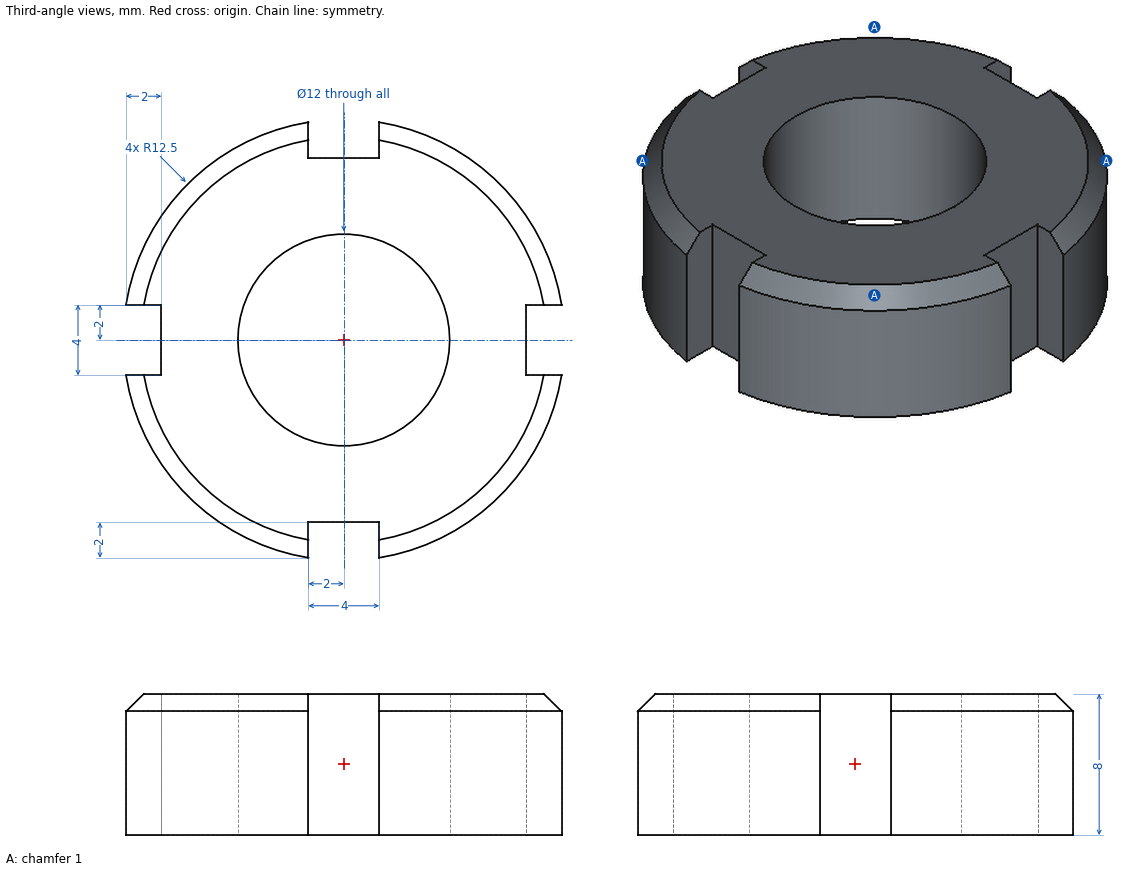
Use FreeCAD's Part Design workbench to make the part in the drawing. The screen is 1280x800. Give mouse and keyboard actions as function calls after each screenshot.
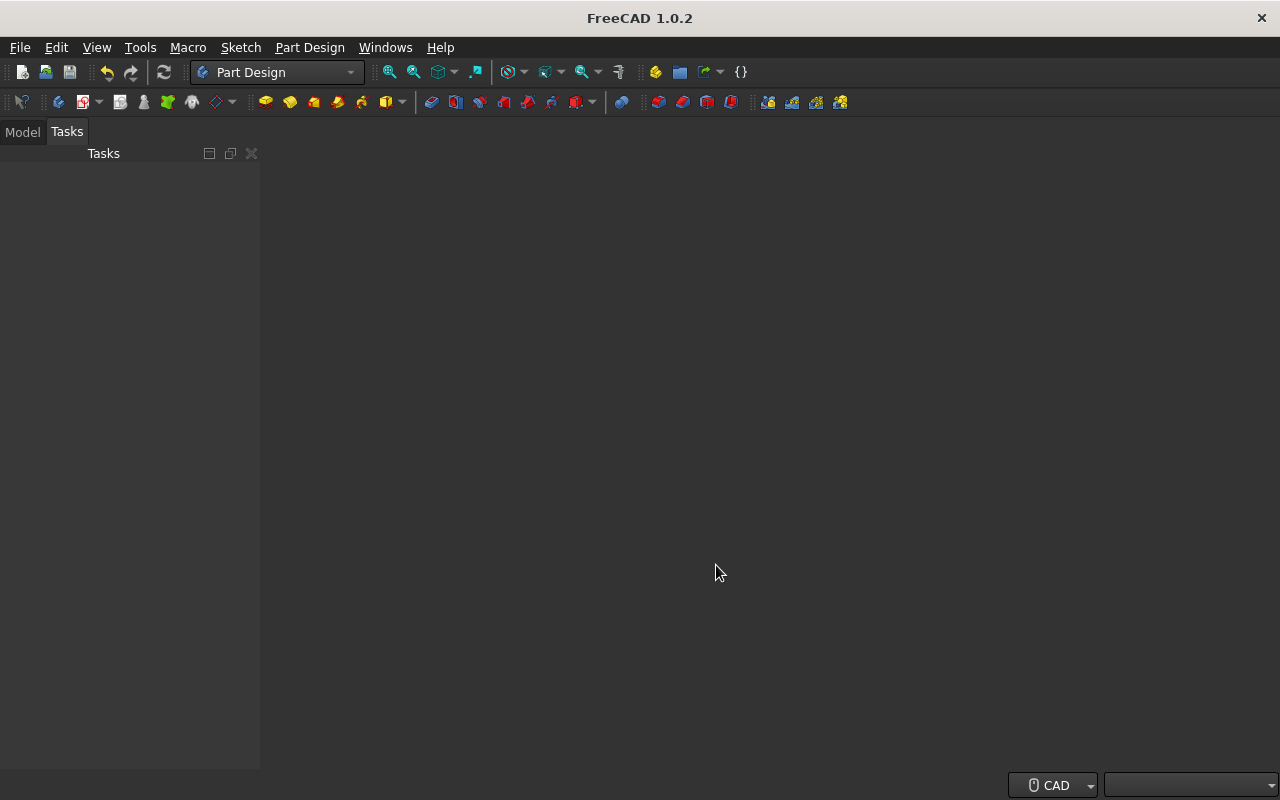
click(22, 72)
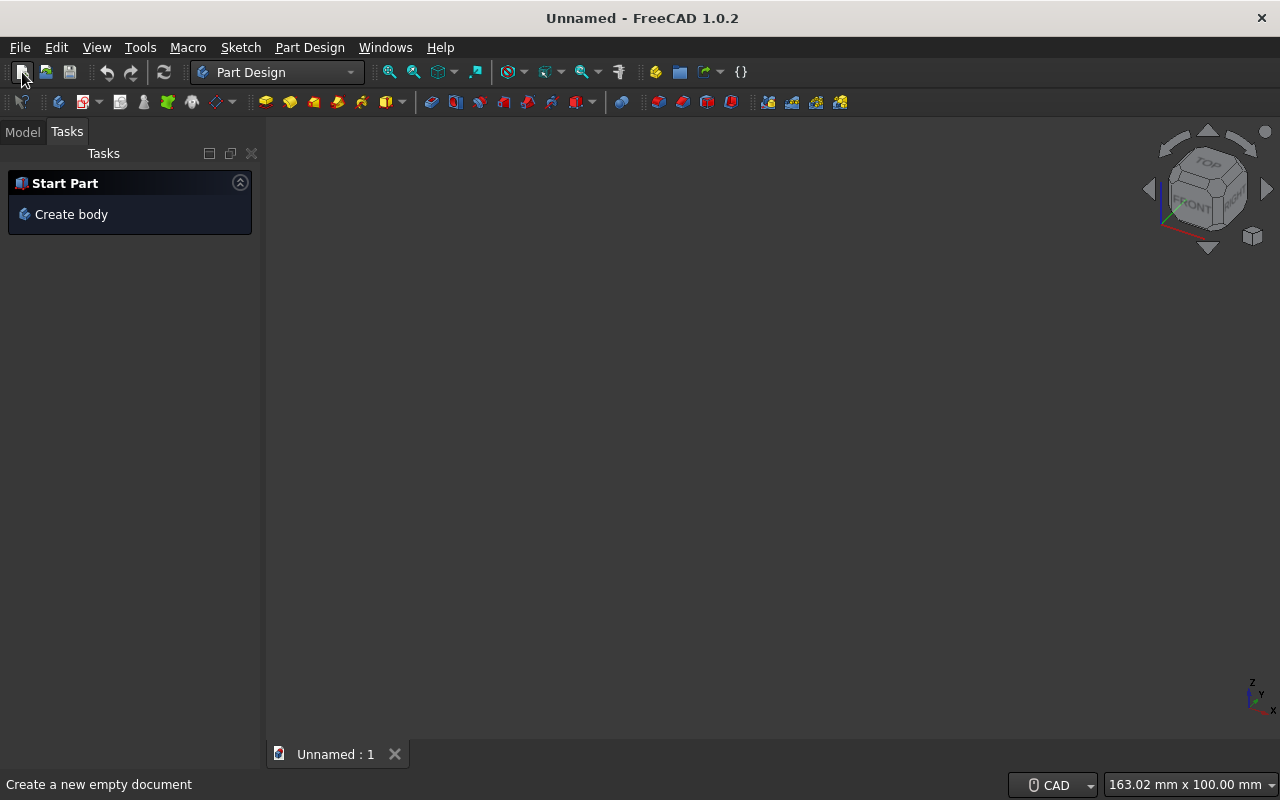
click(84, 102)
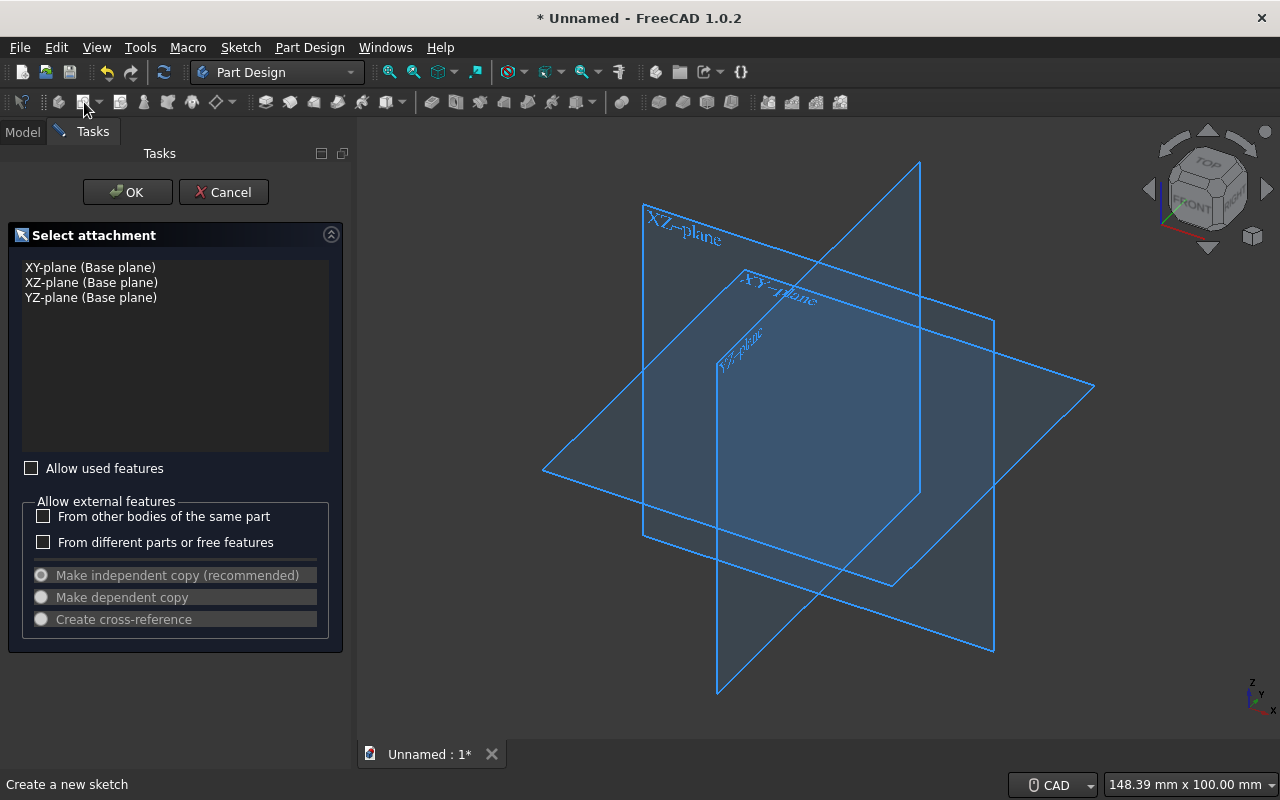
click(82, 268)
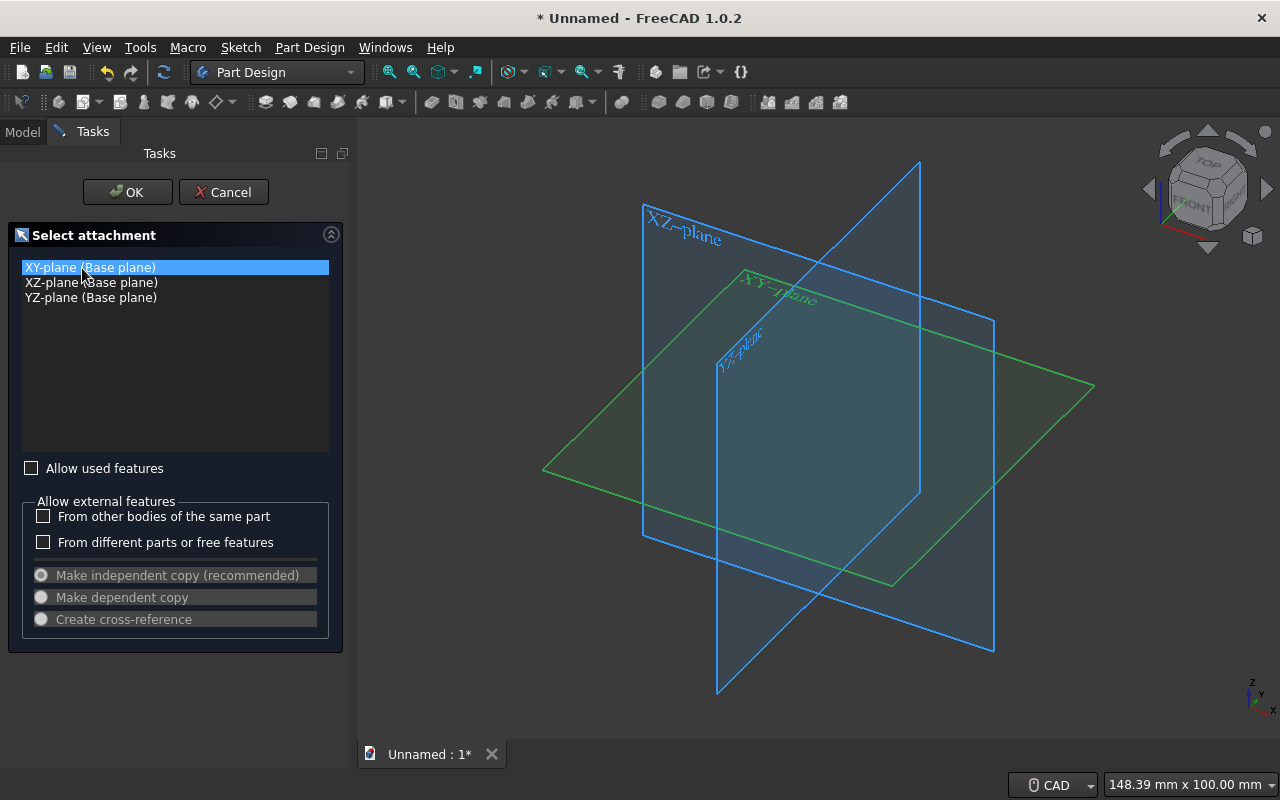
click(128, 192)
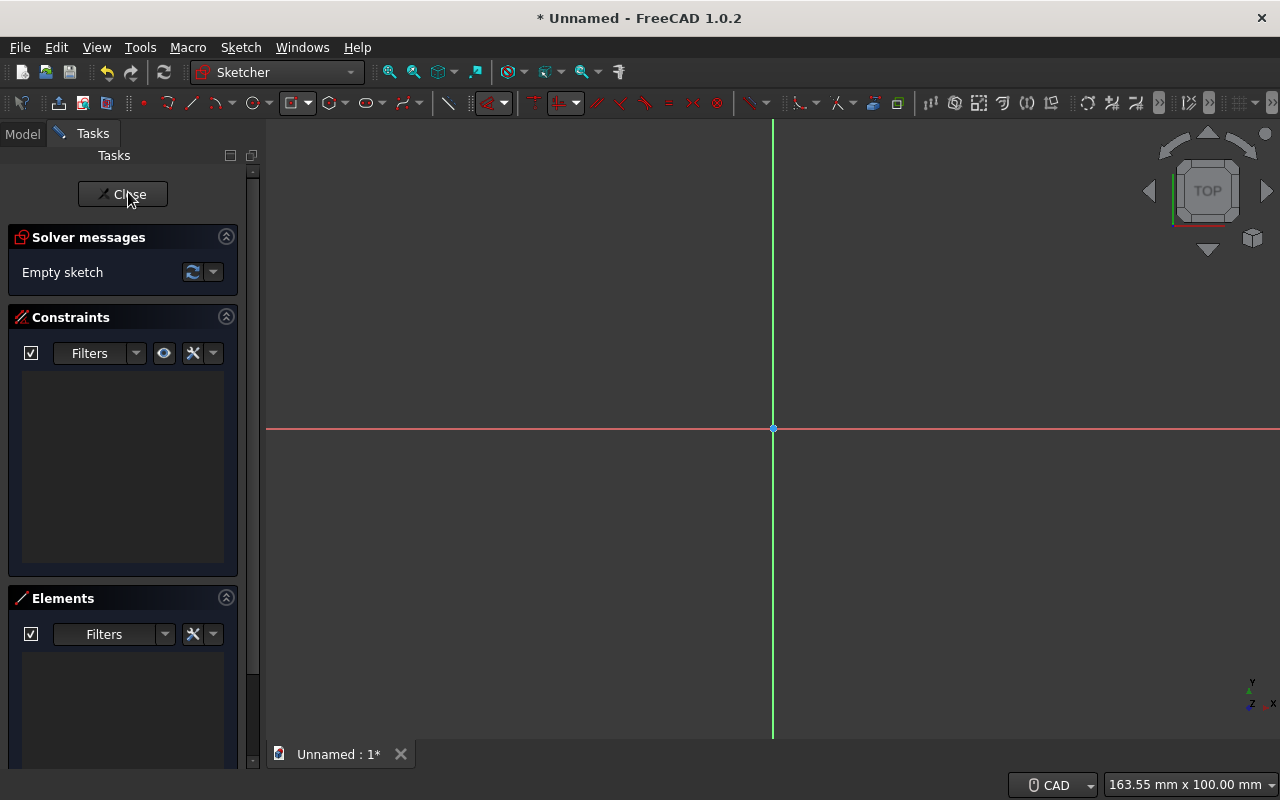
scroll(813, 429, up, 5)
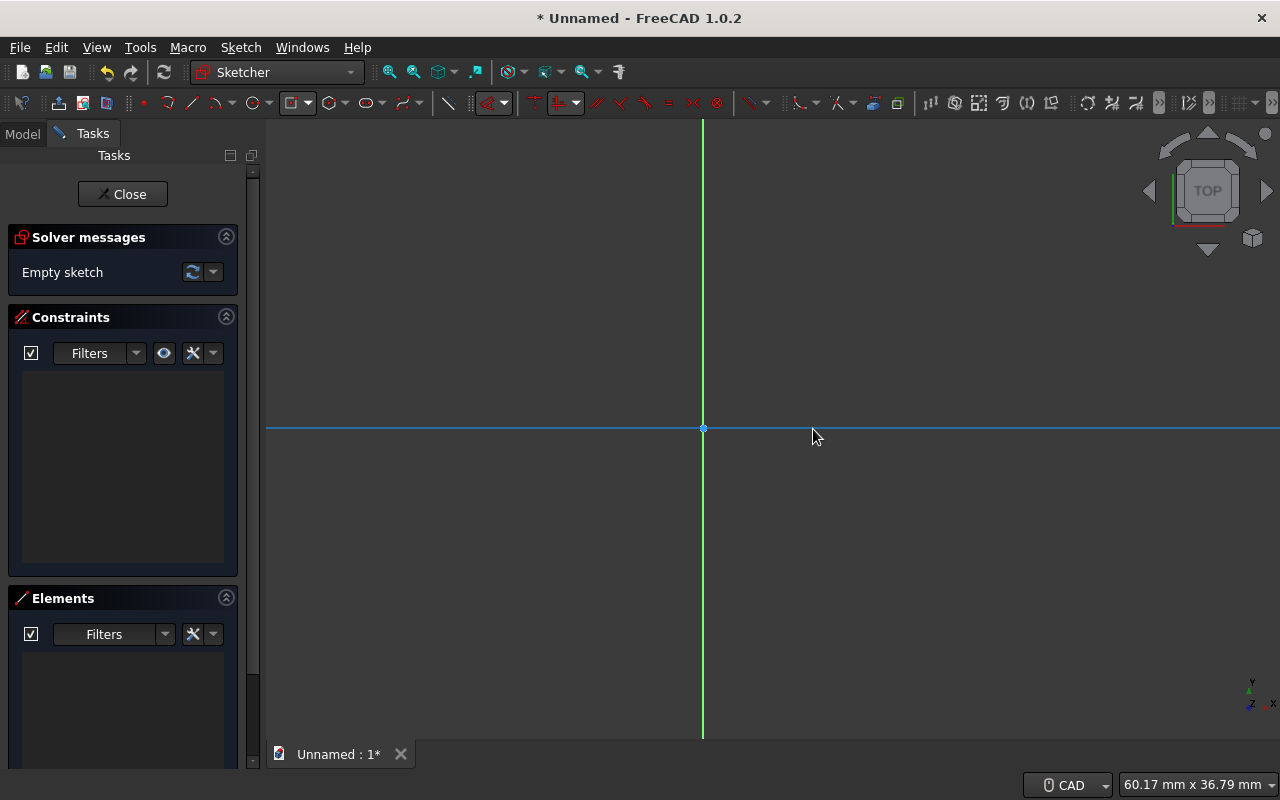
key(g)
key(m)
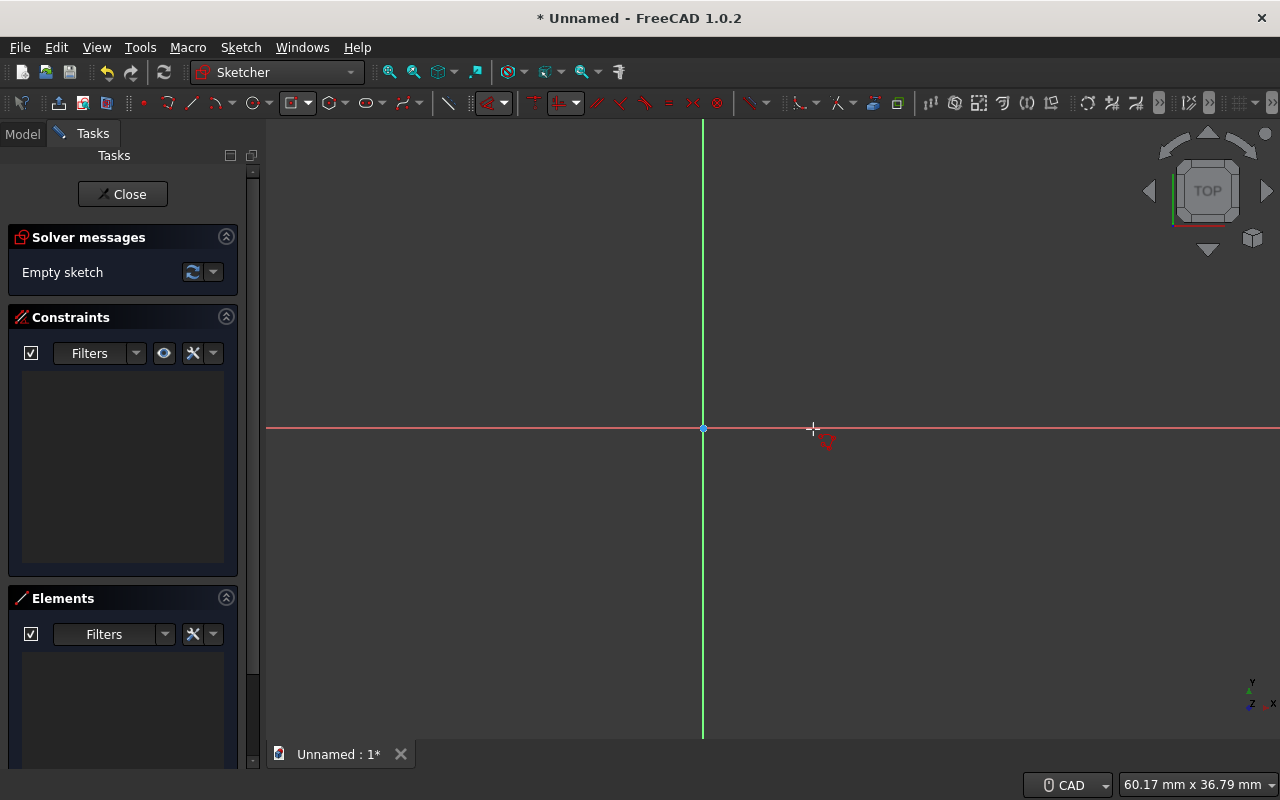
click(495, 394)
click(529, 394)
click(529, 462)
click(495, 462)
right_click(495, 462)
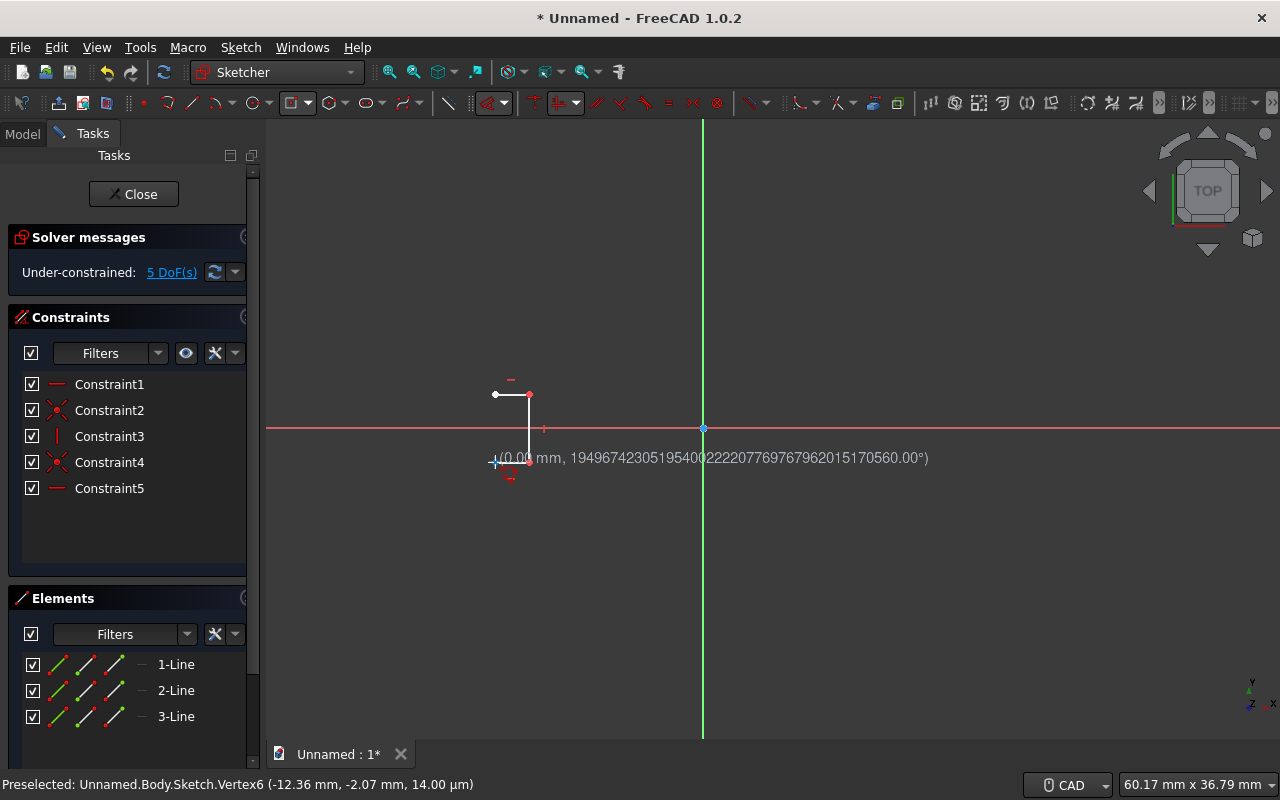
click(670, 636)
click(670, 602)
click(737, 602)
click(737, 636)
right_click(737, 636)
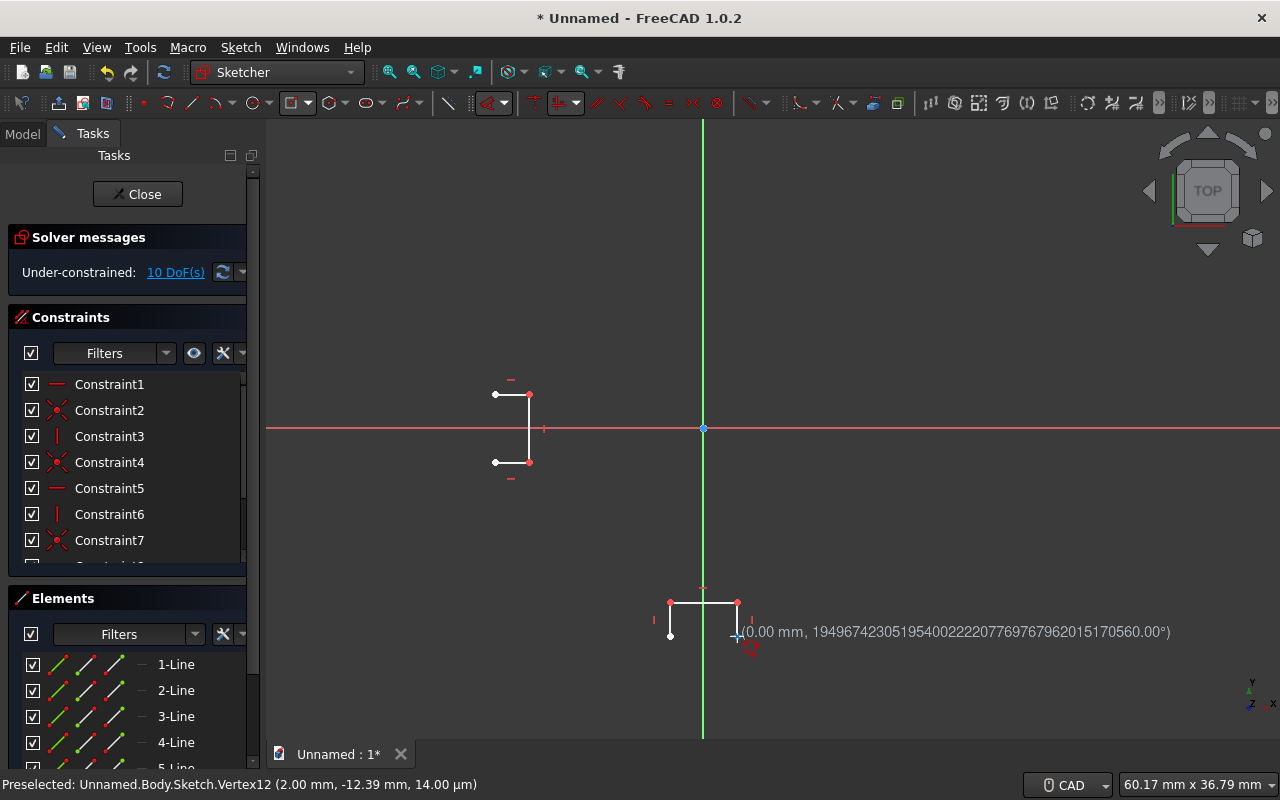
click(911, 462)
click(878, 462)
click(878, 394)
click(911, 394)
right_click(911, 394)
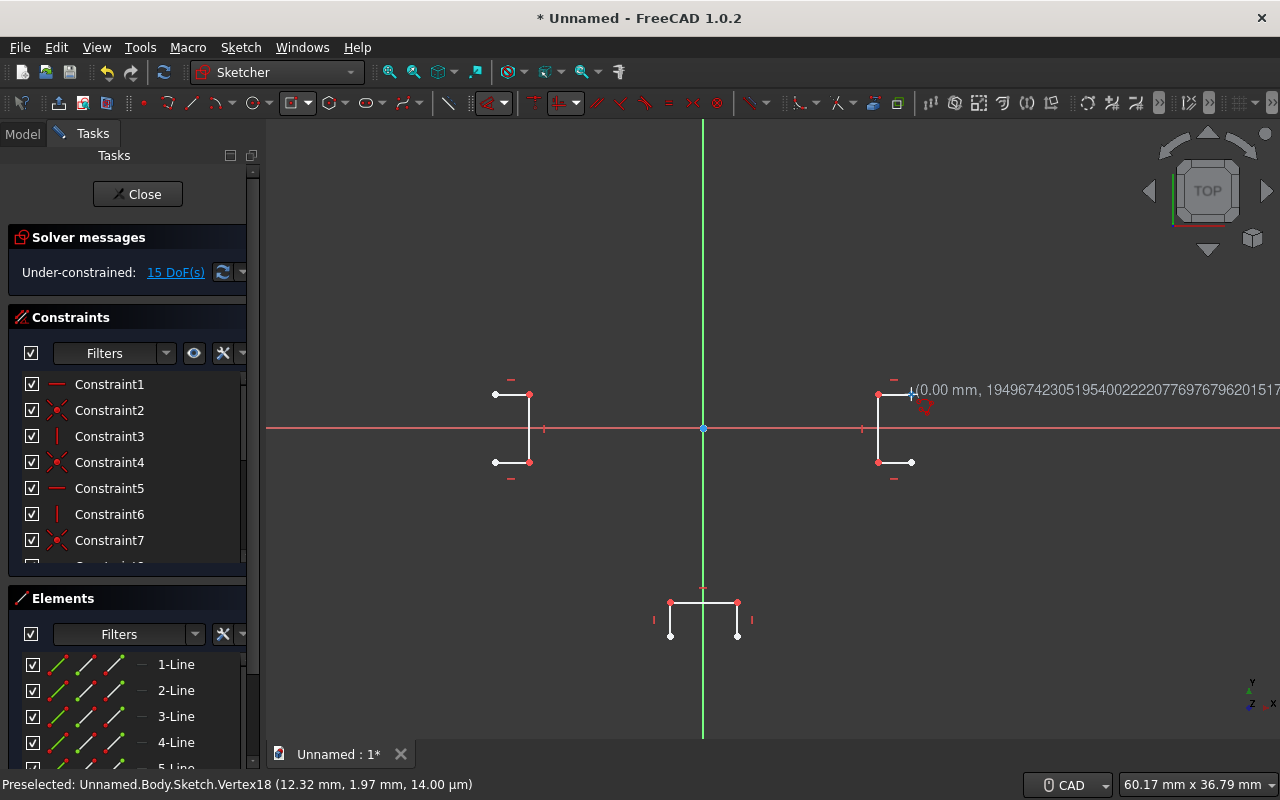
click(737, 220)
click(737, 254)
click(670, 254)
click(670, 220)
right_click(670, 220)